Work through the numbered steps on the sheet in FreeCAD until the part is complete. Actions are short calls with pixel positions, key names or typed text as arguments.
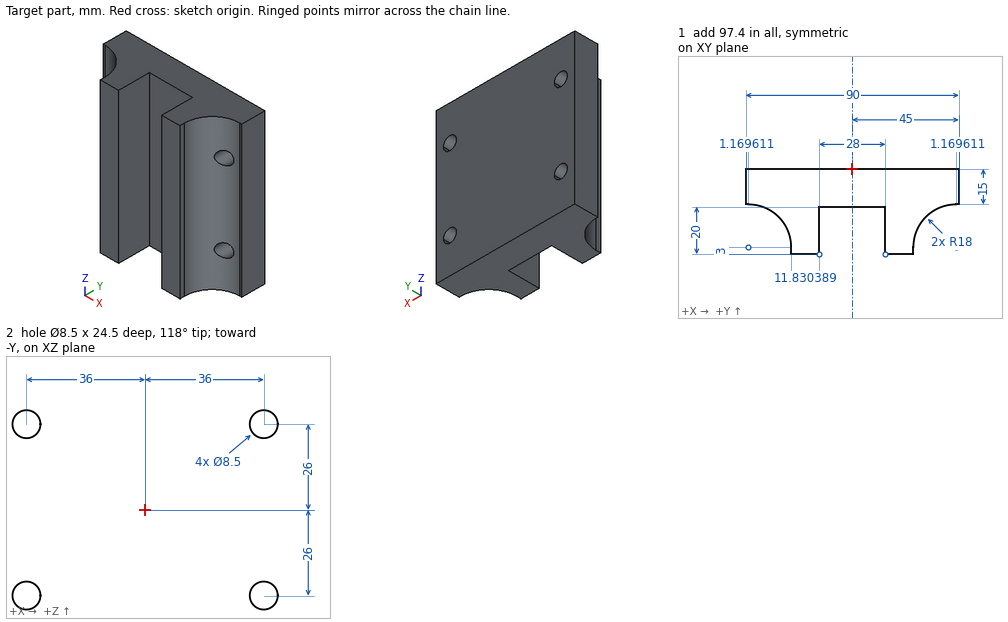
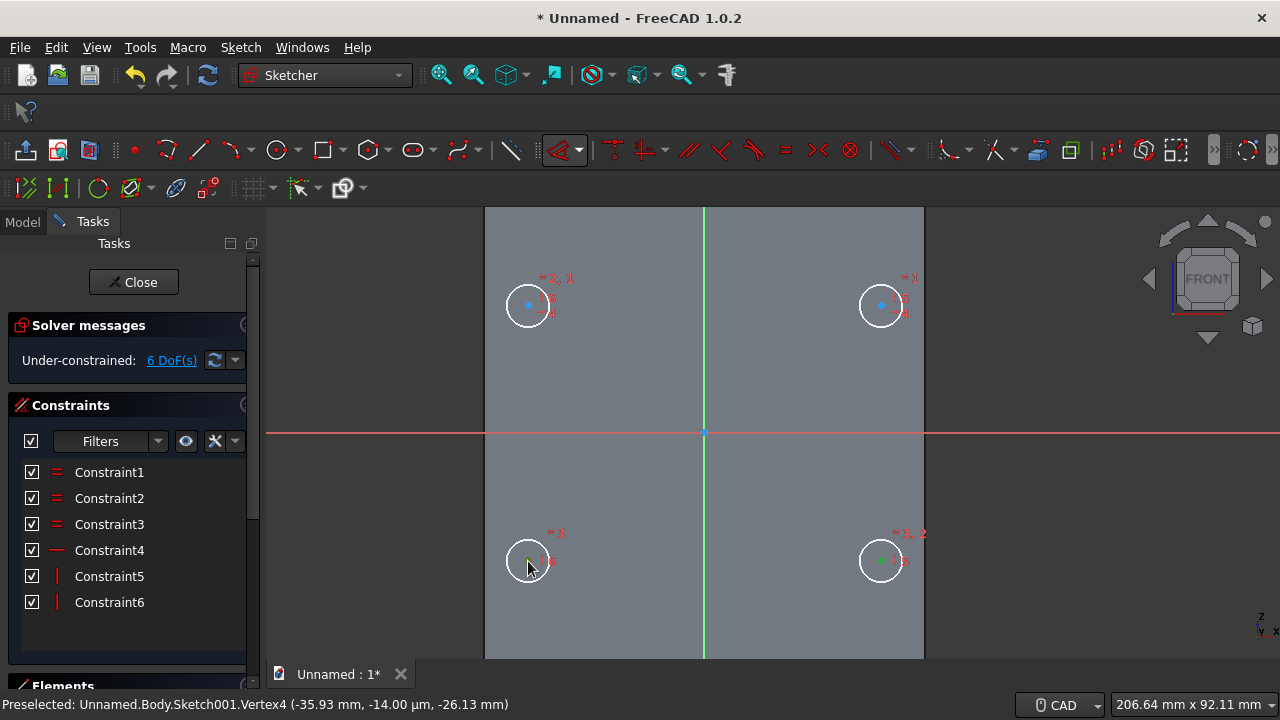
key(h)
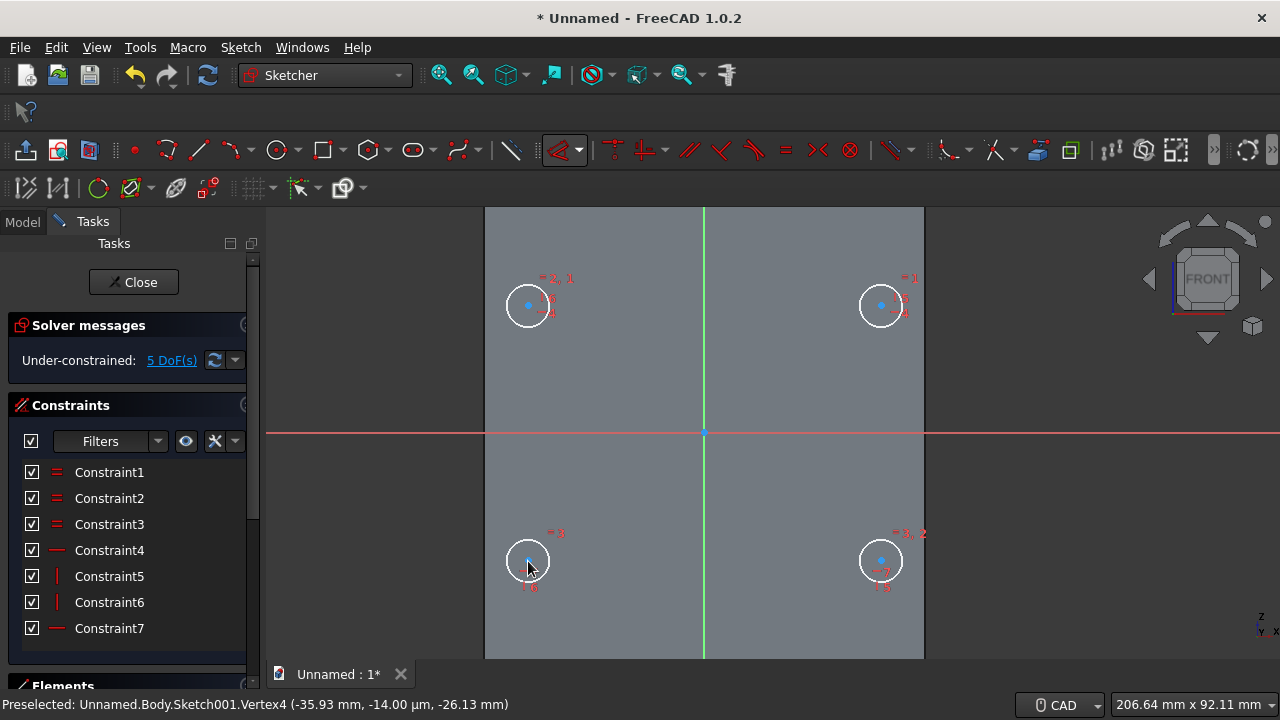
click(866, 291)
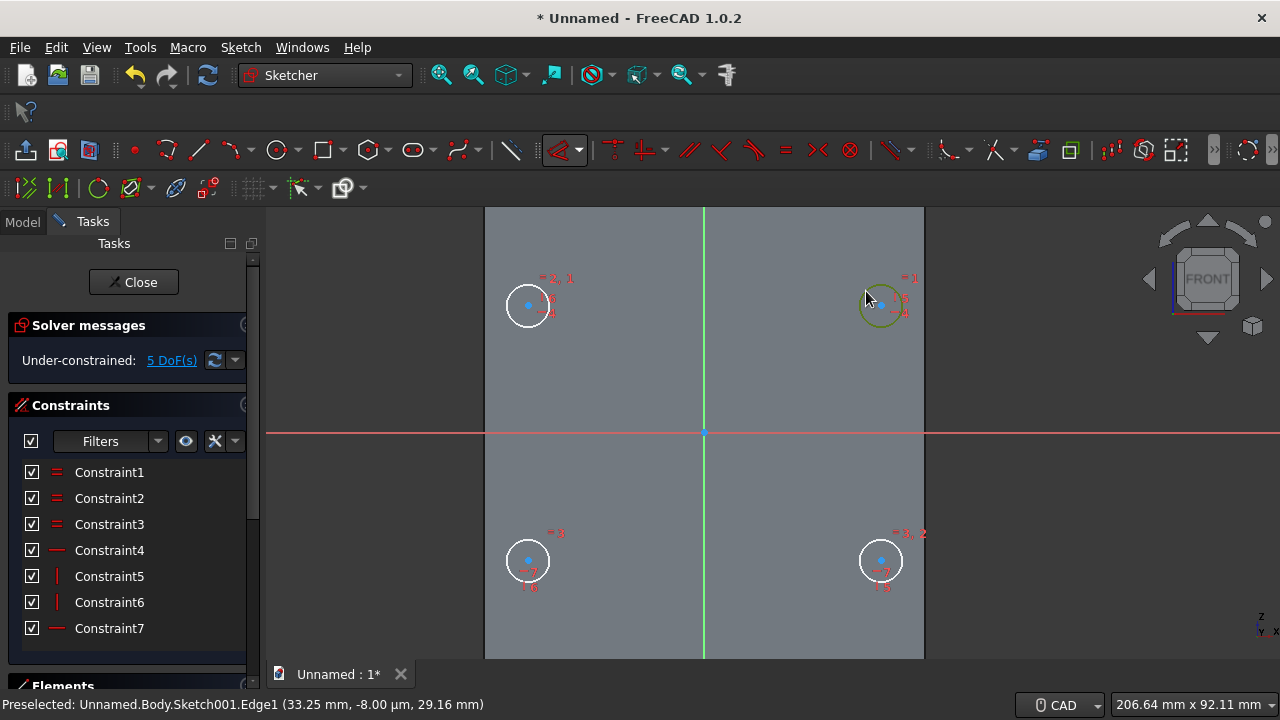
key(k)
key(o)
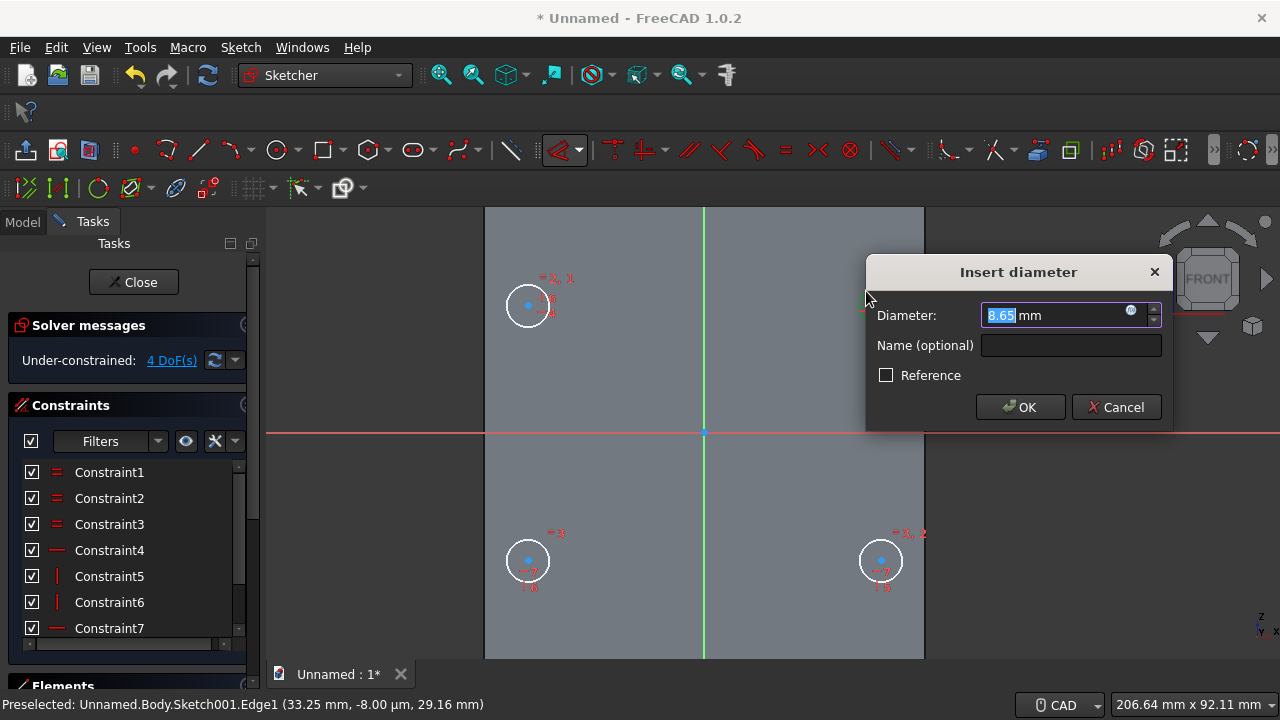
text(8.5)
key(Return)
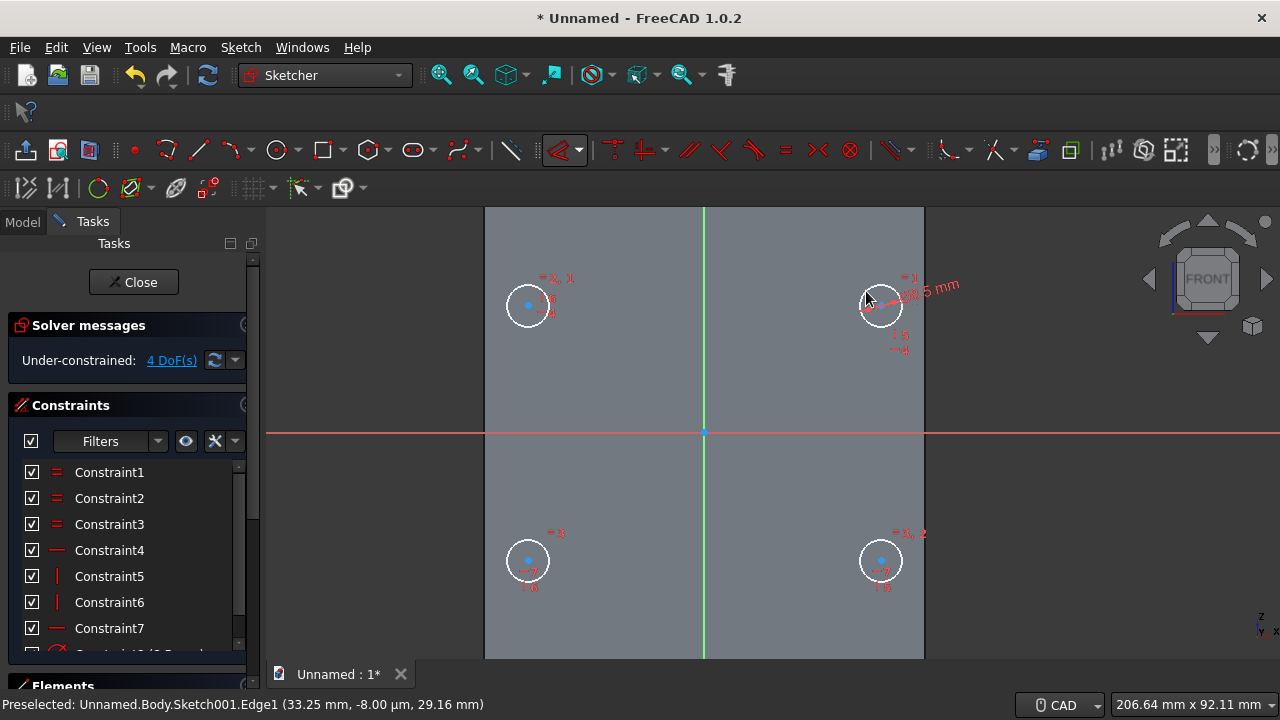
click(881, 306)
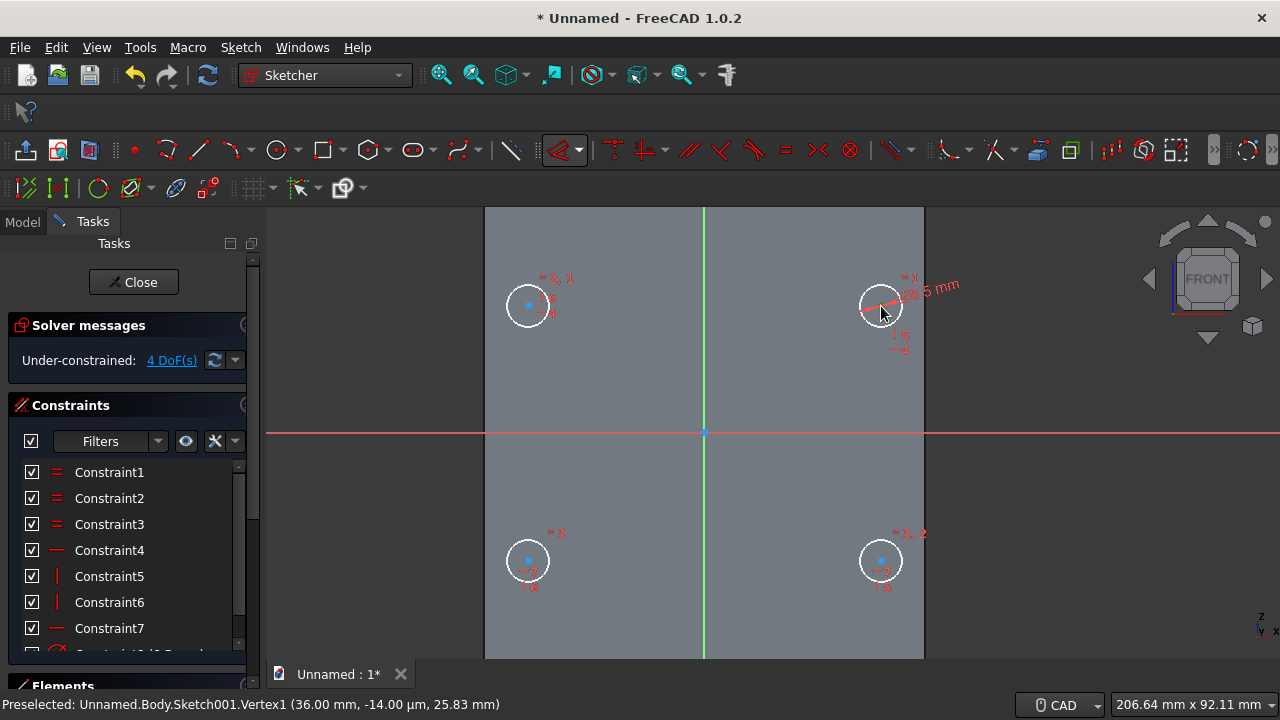
click(582, 150)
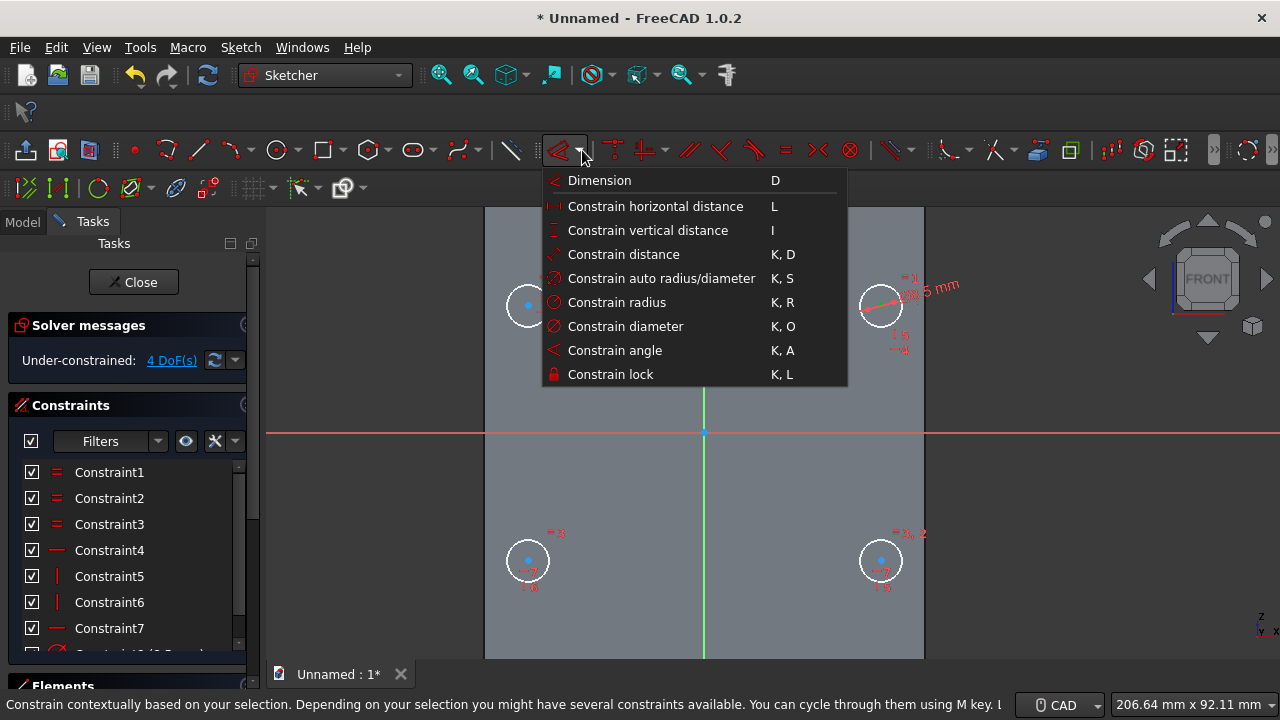
click(695, 206)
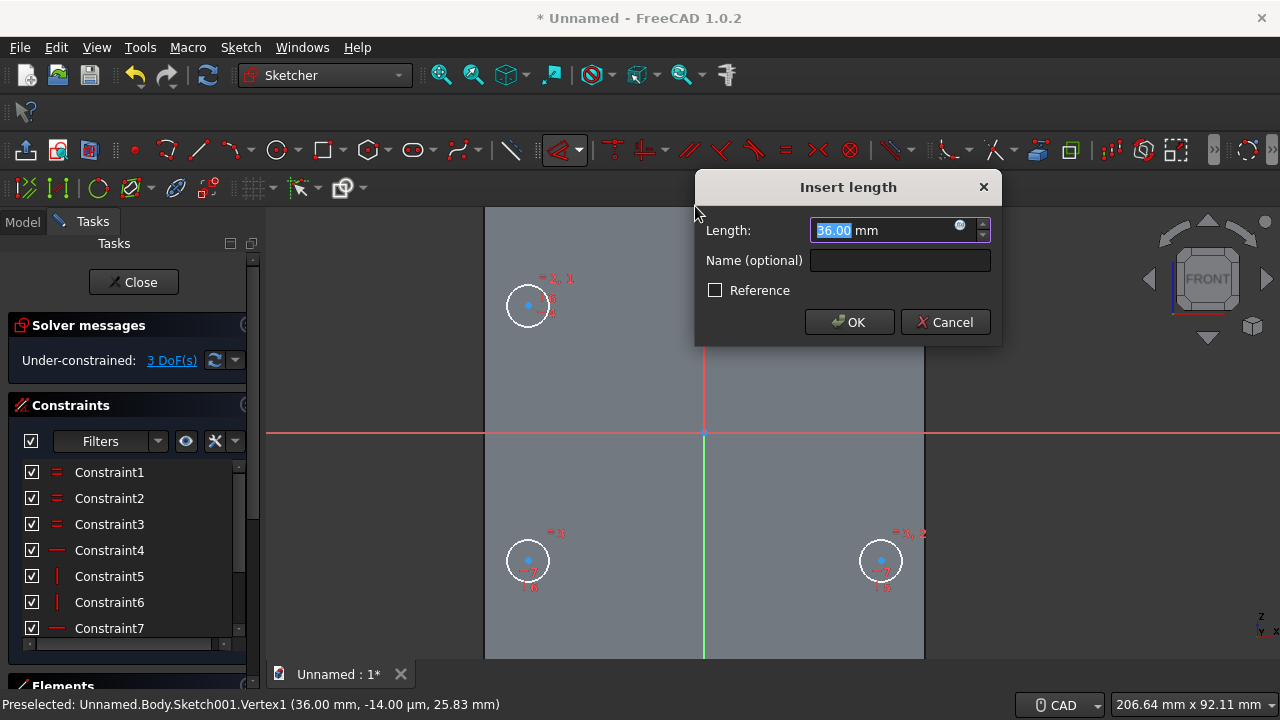
text(36)
key(Return)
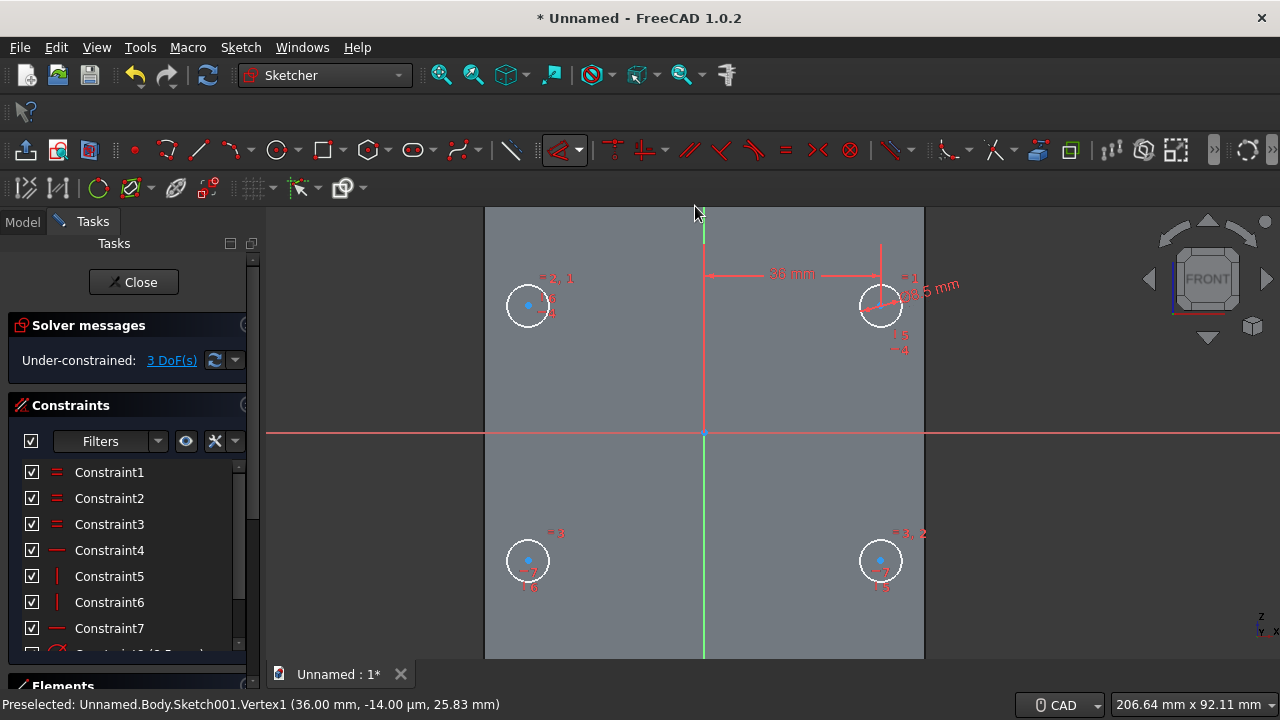
click(881, 306)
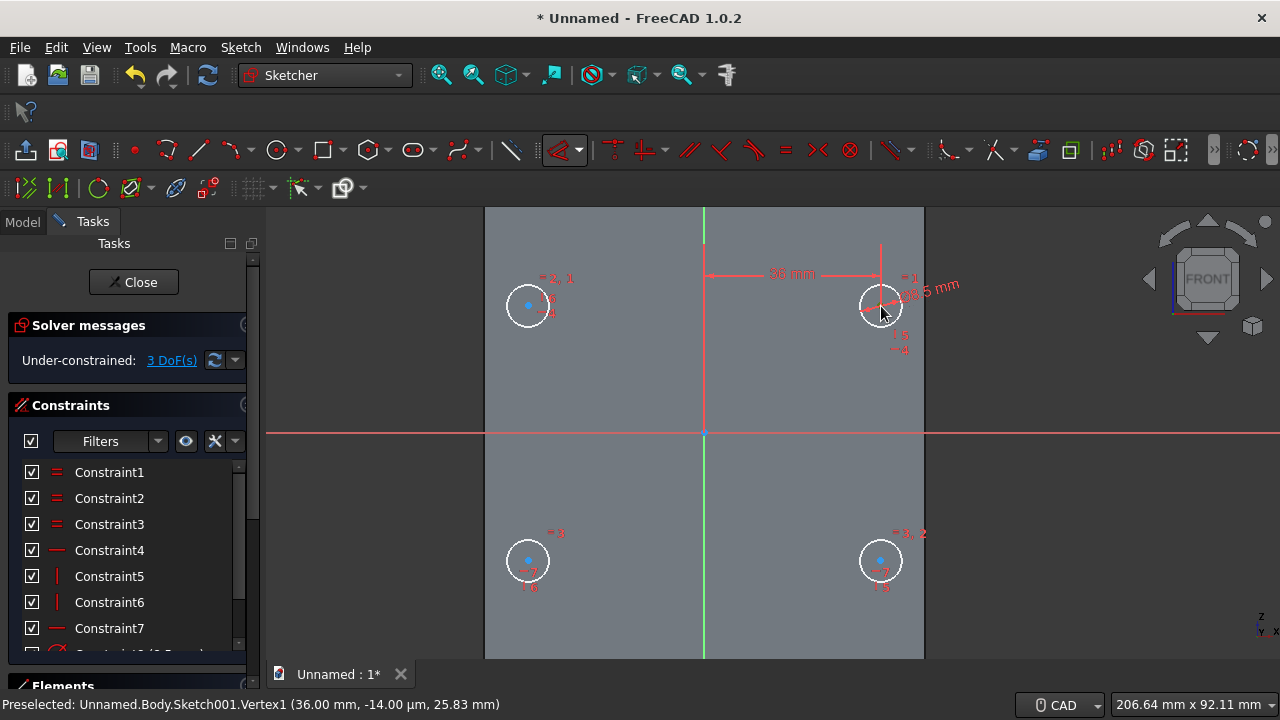
key(i)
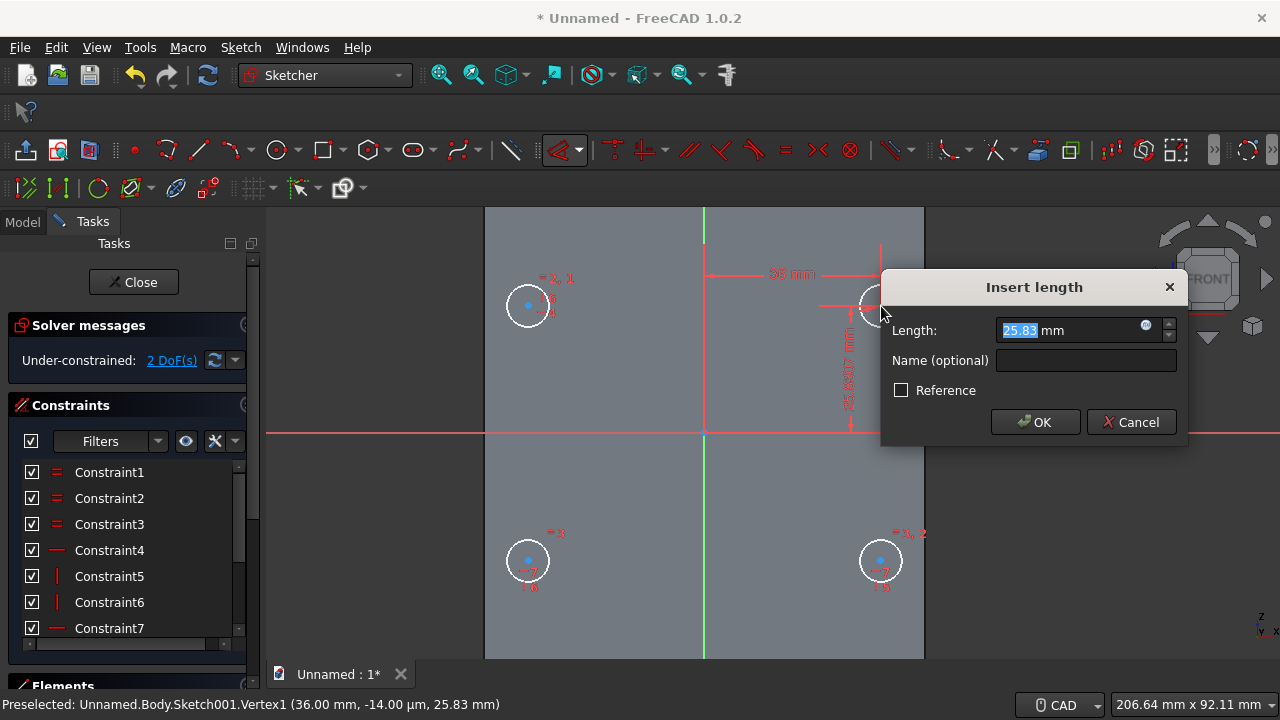
text(26)
key(Return)